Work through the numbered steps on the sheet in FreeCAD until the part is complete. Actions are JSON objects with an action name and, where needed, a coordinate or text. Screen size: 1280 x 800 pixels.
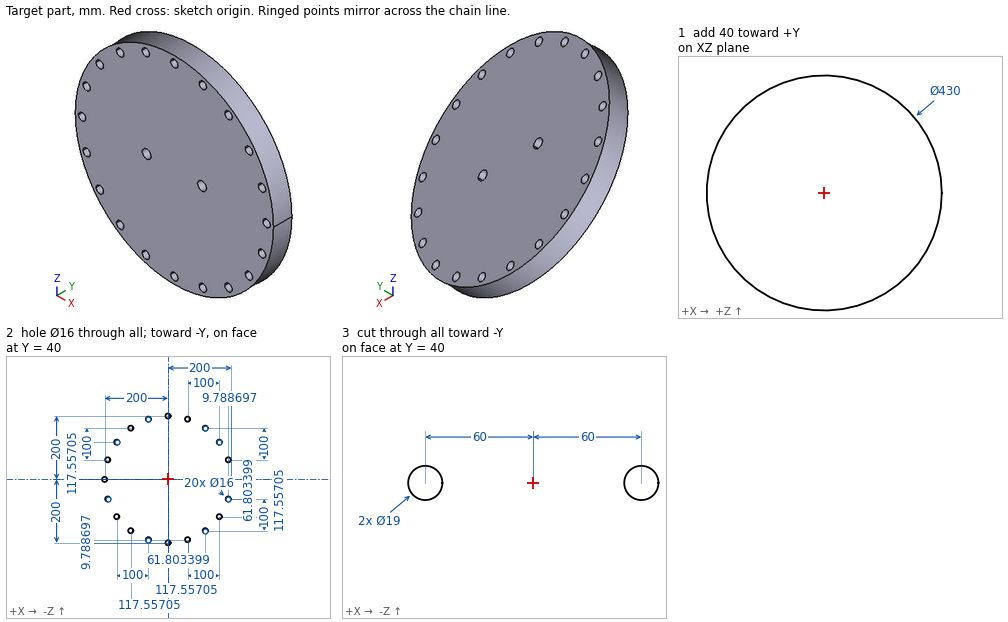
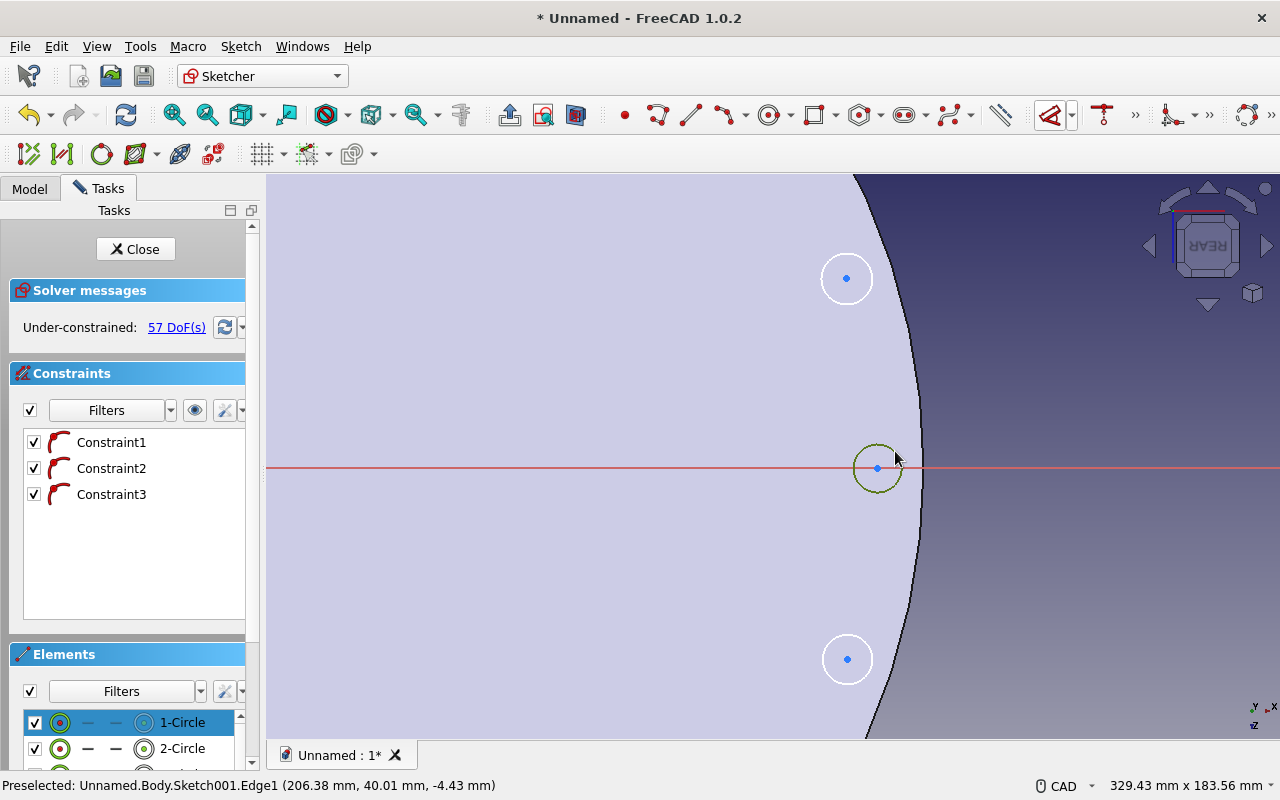
{"action": "left_click", "coordinate": [865, 642]}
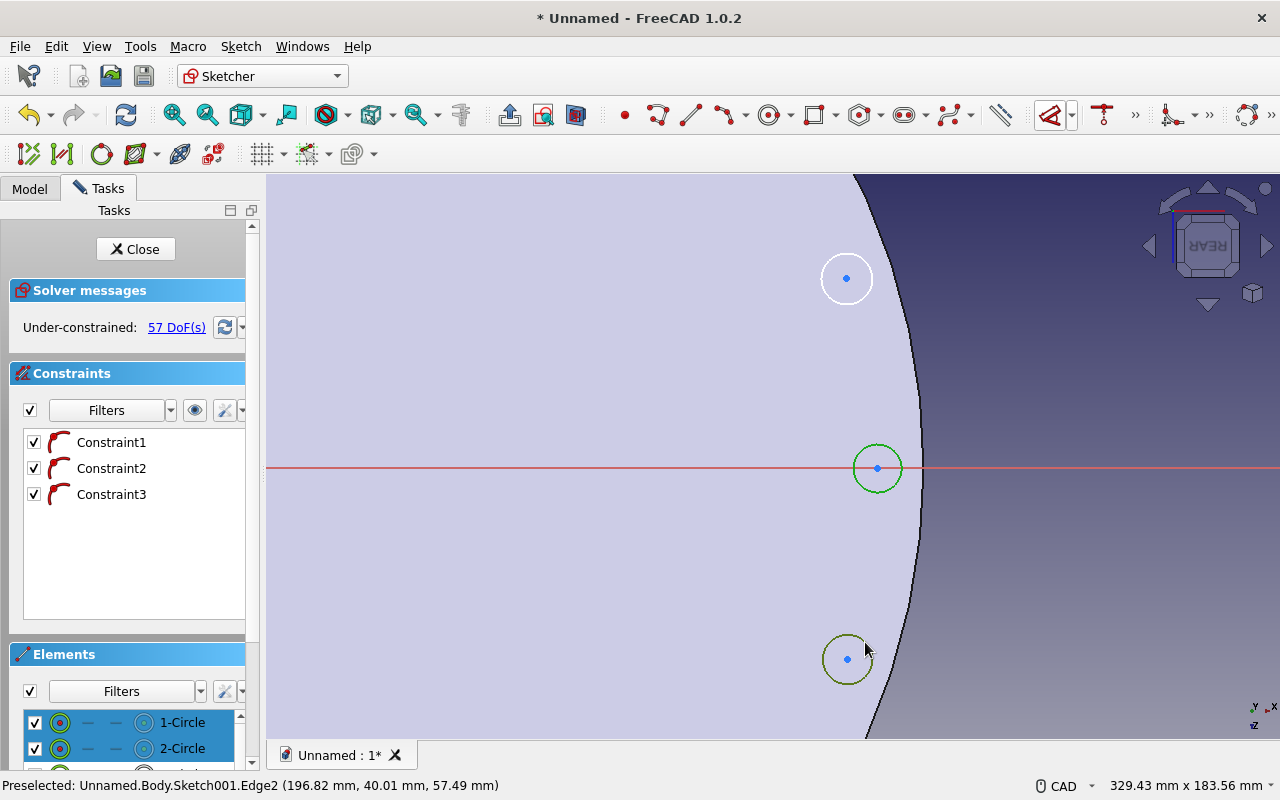
{"action": "scroll", "coordinate": [895, 452], "scroll_direction": "down", "scroll_amount": 6}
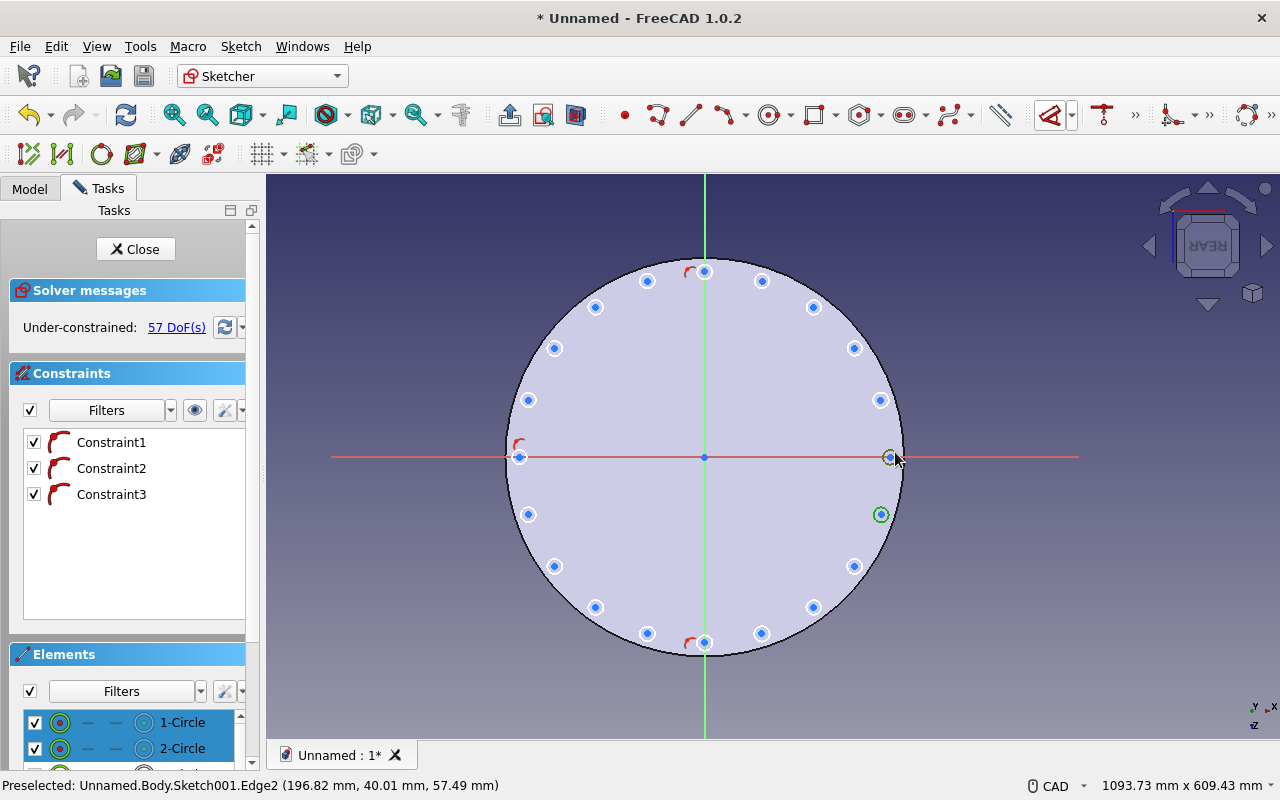
{"action": "scroll", "coordinate": [860, 561], "scroll_direction": "up", "scroll_amount": 4}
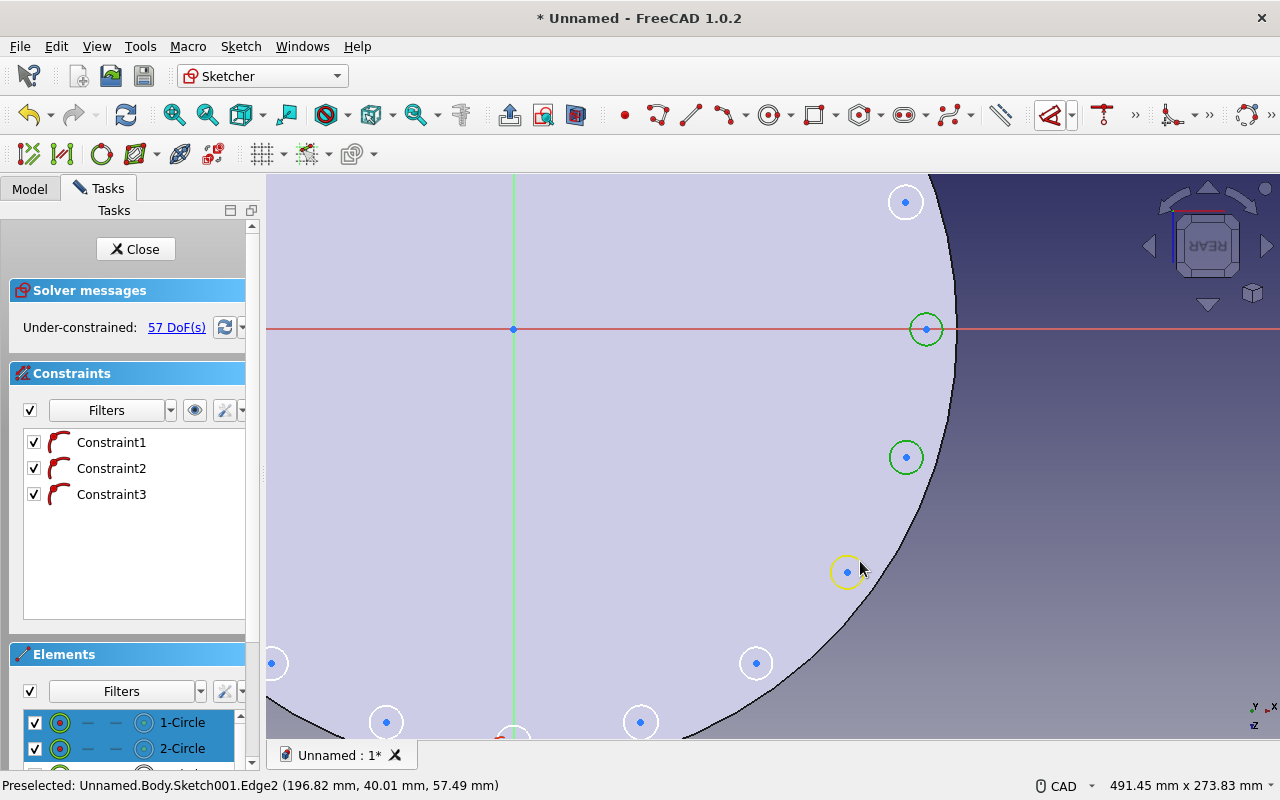
{"action": "left_click", "coordinate": [859, 561]}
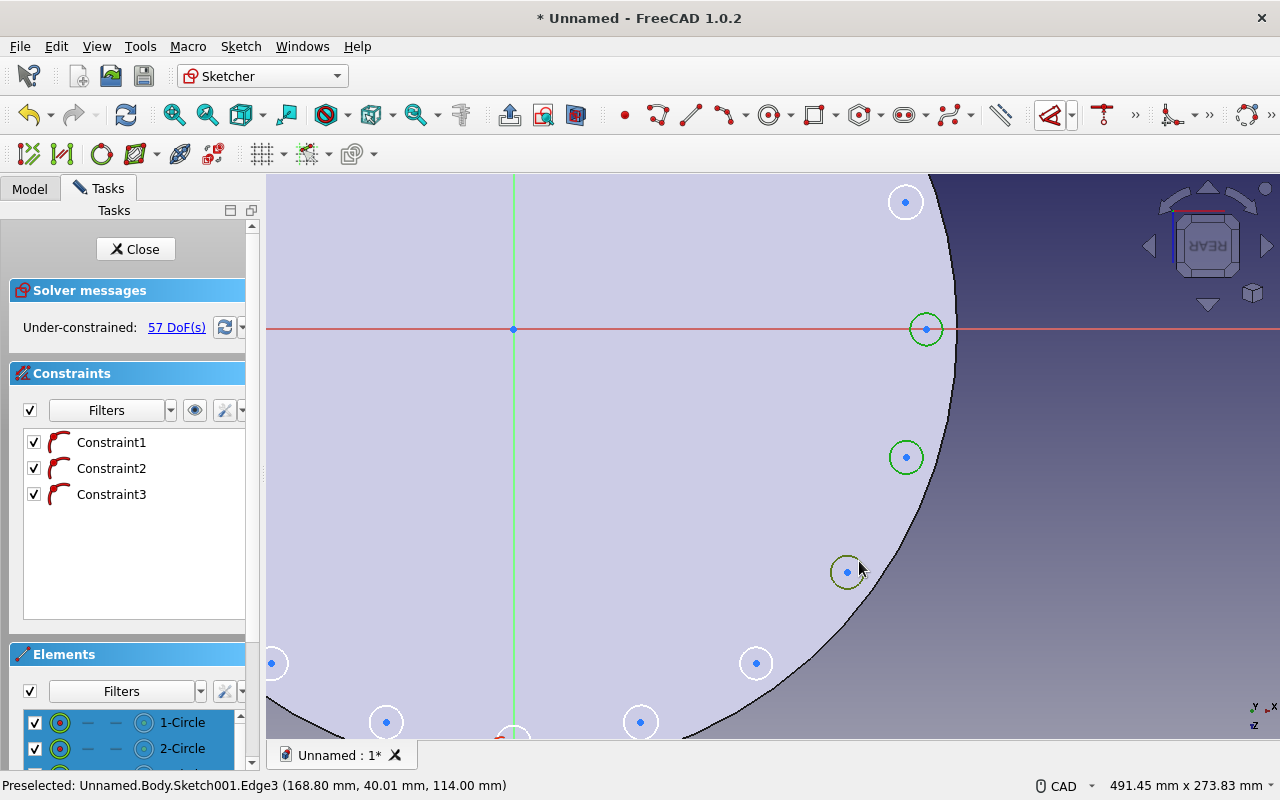
{"action": "left_click", "coordinate": [768, 652]}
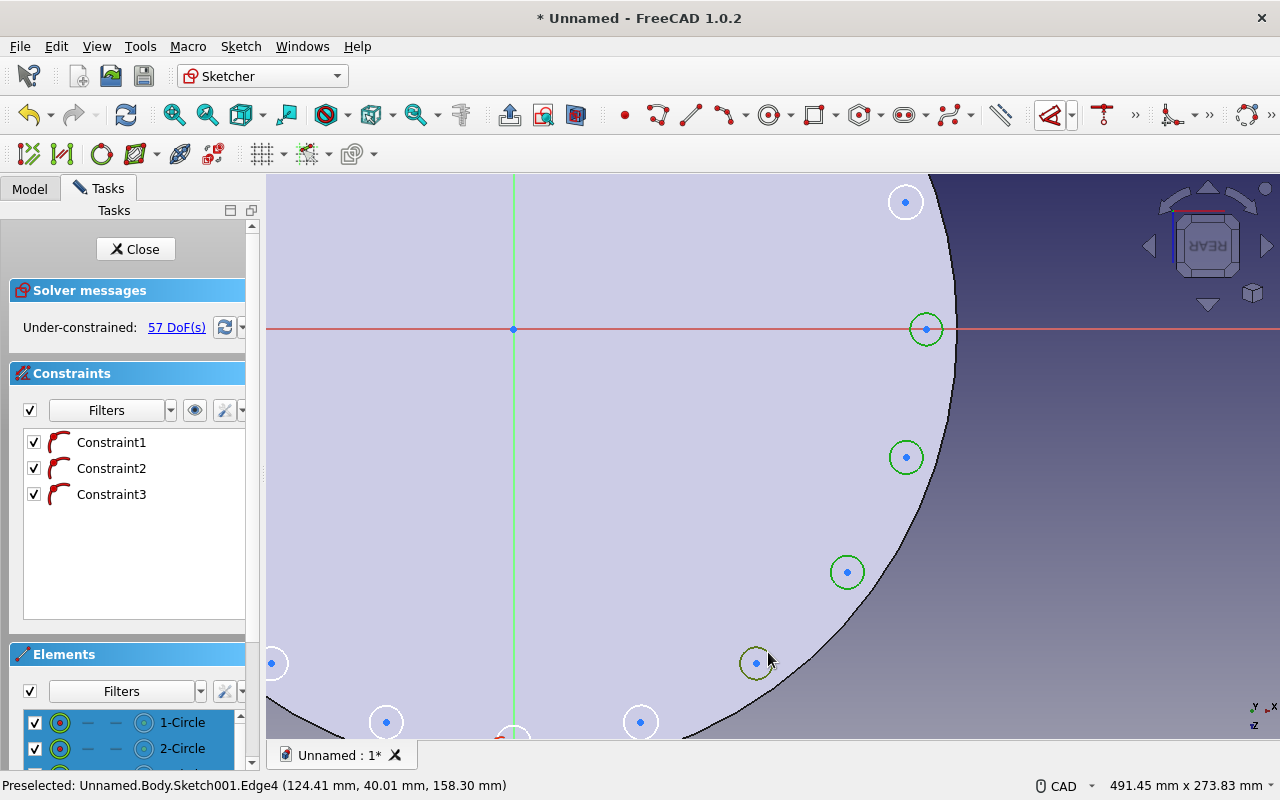
{"action": "left_click", "coordinate": [653, 710]}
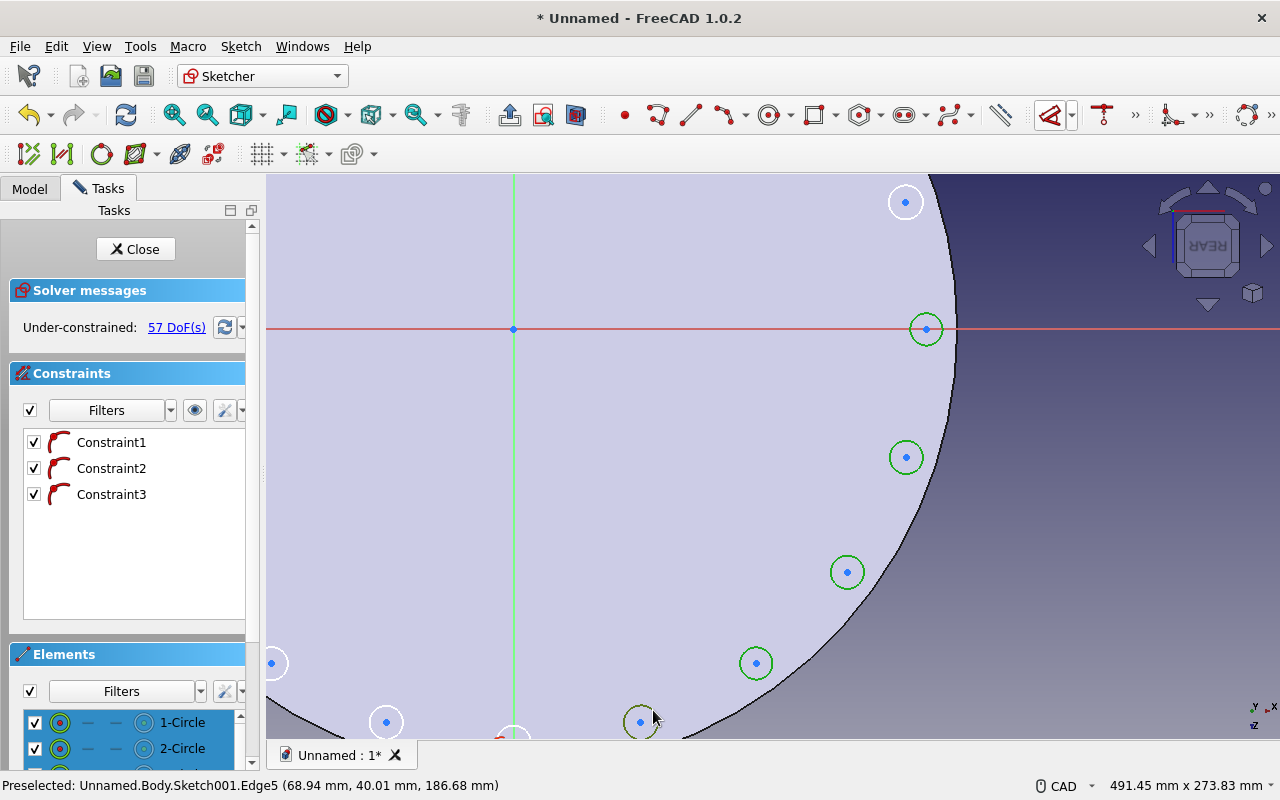
{"action": "scroll", "coordinate": [860, 560], "scroll_direction": "down", "scroll_amount": 4}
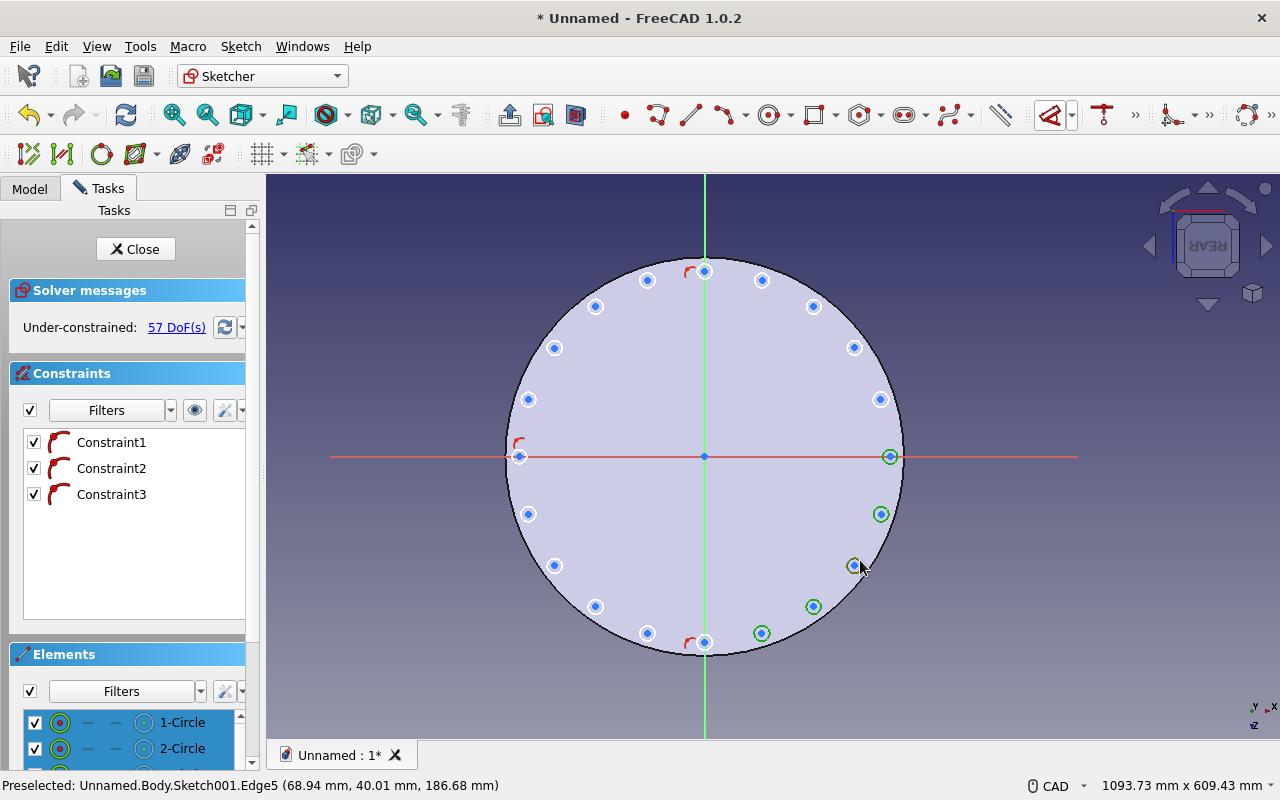
{"action": "scroll", "coordinate": [710, 637], "scroll_direction": "up", "scroll_amount": 5}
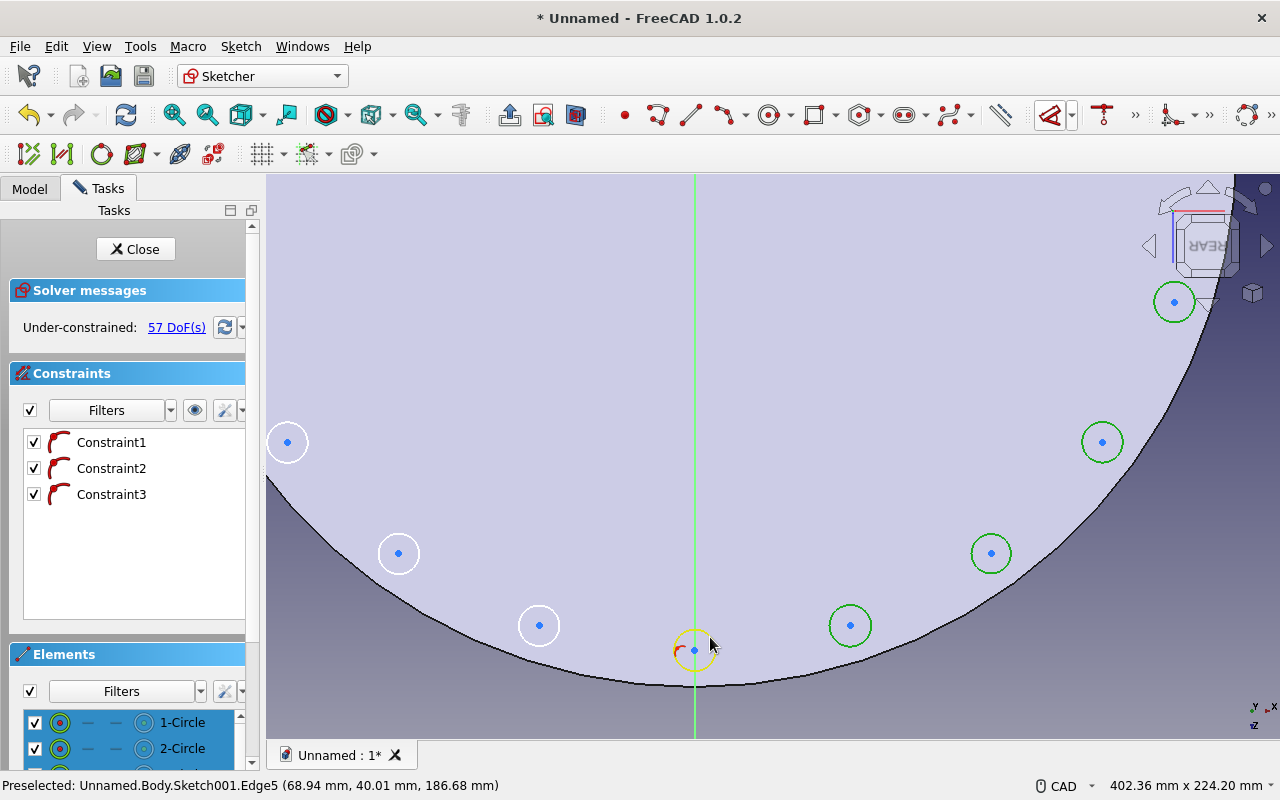
{"action": "left_click", "coordinate": [710, 636]}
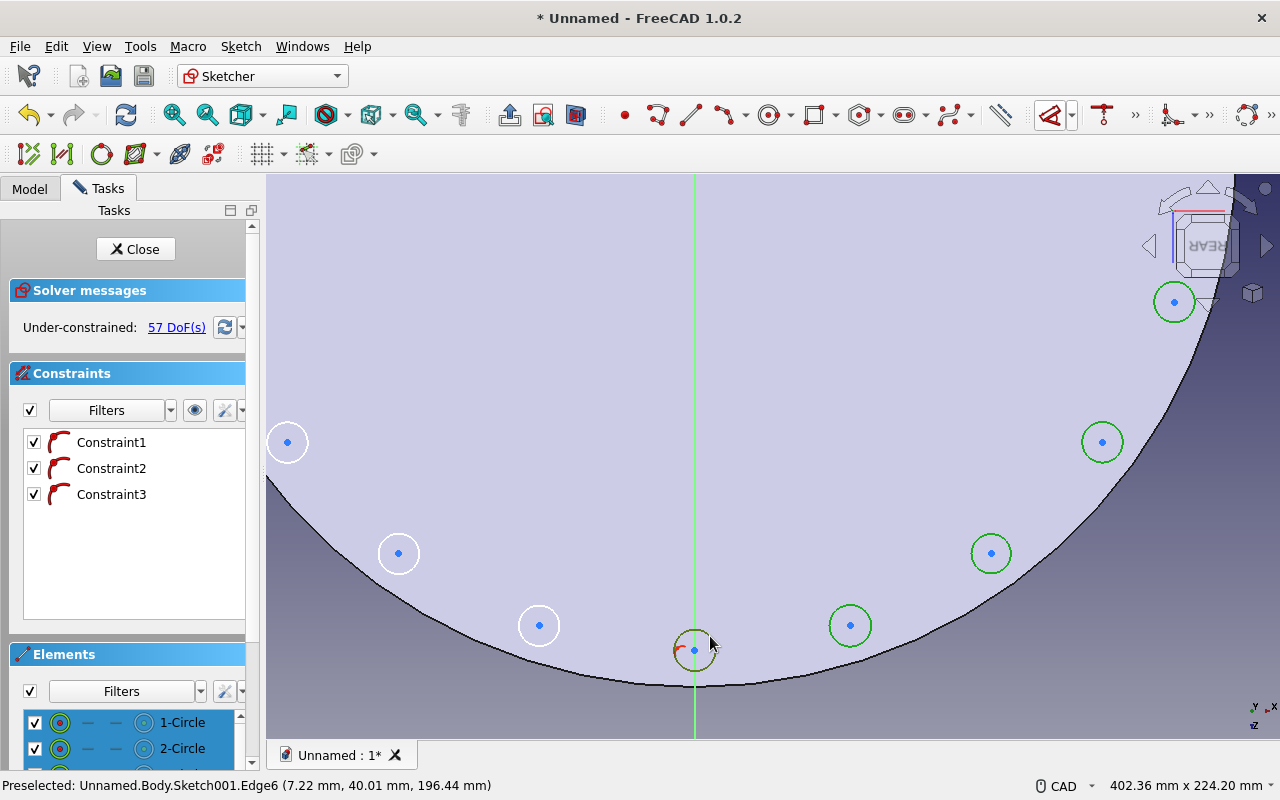
{"action": "left_click", "coordinate": [554, 611]}